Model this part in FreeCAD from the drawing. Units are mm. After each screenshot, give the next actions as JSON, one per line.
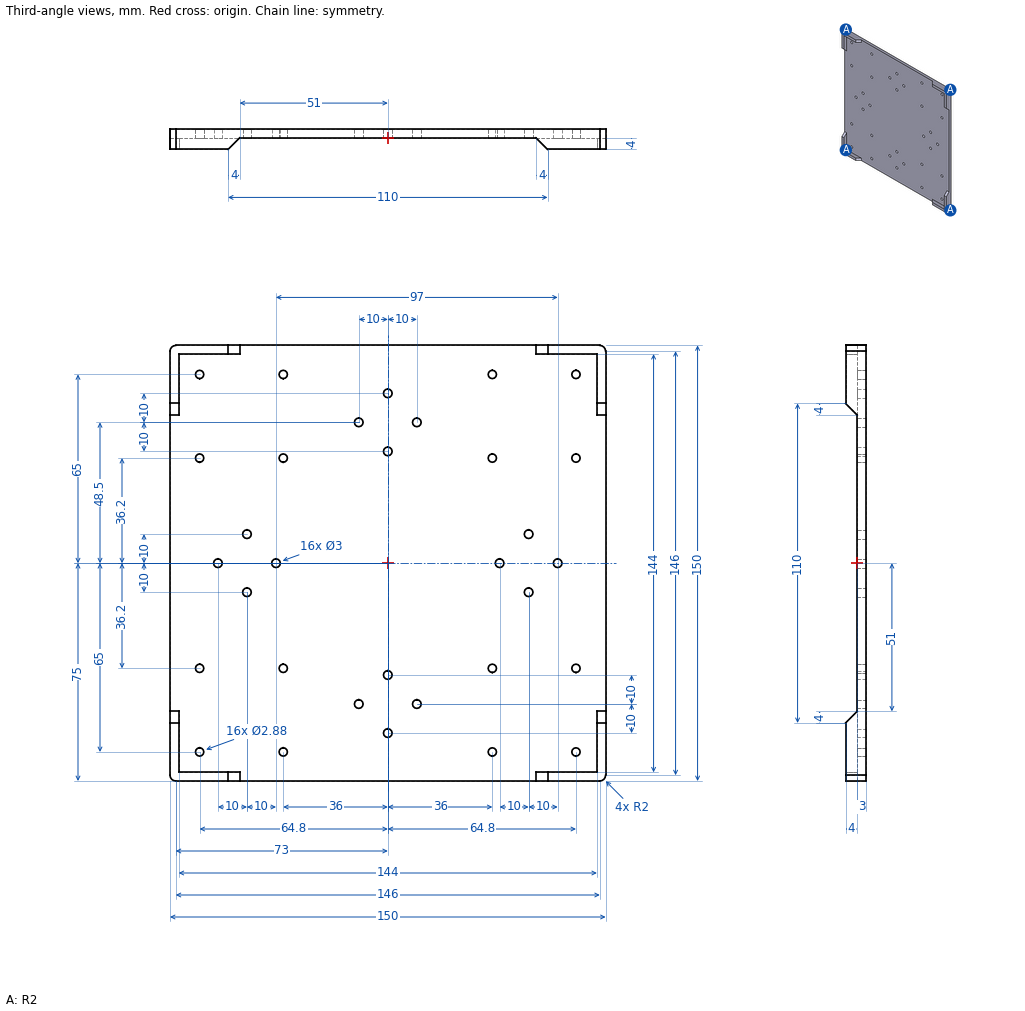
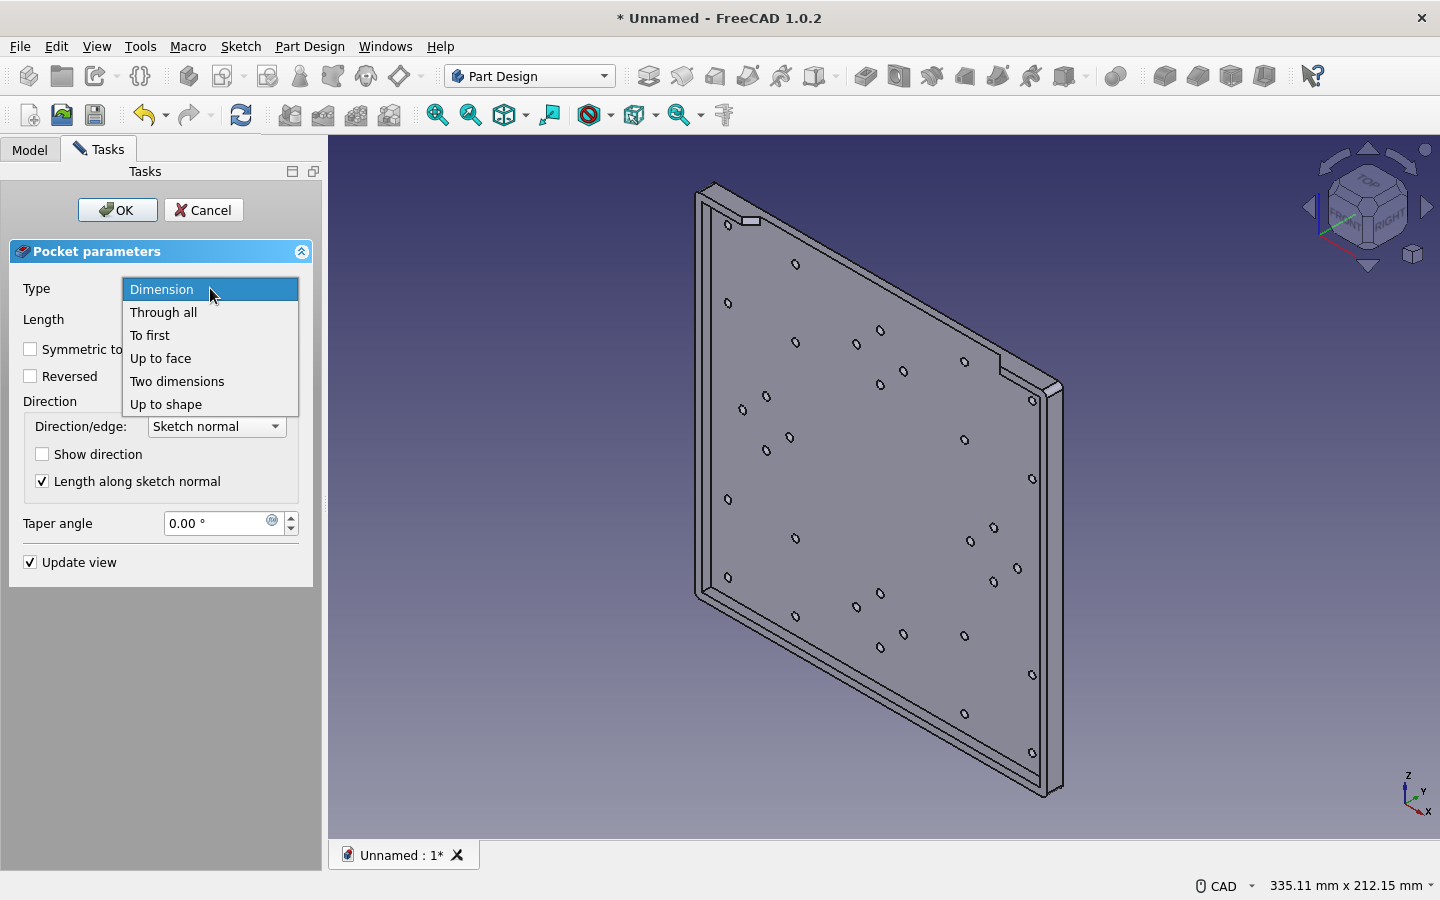
{"action": "left_click", "coordinate": [208, 312]}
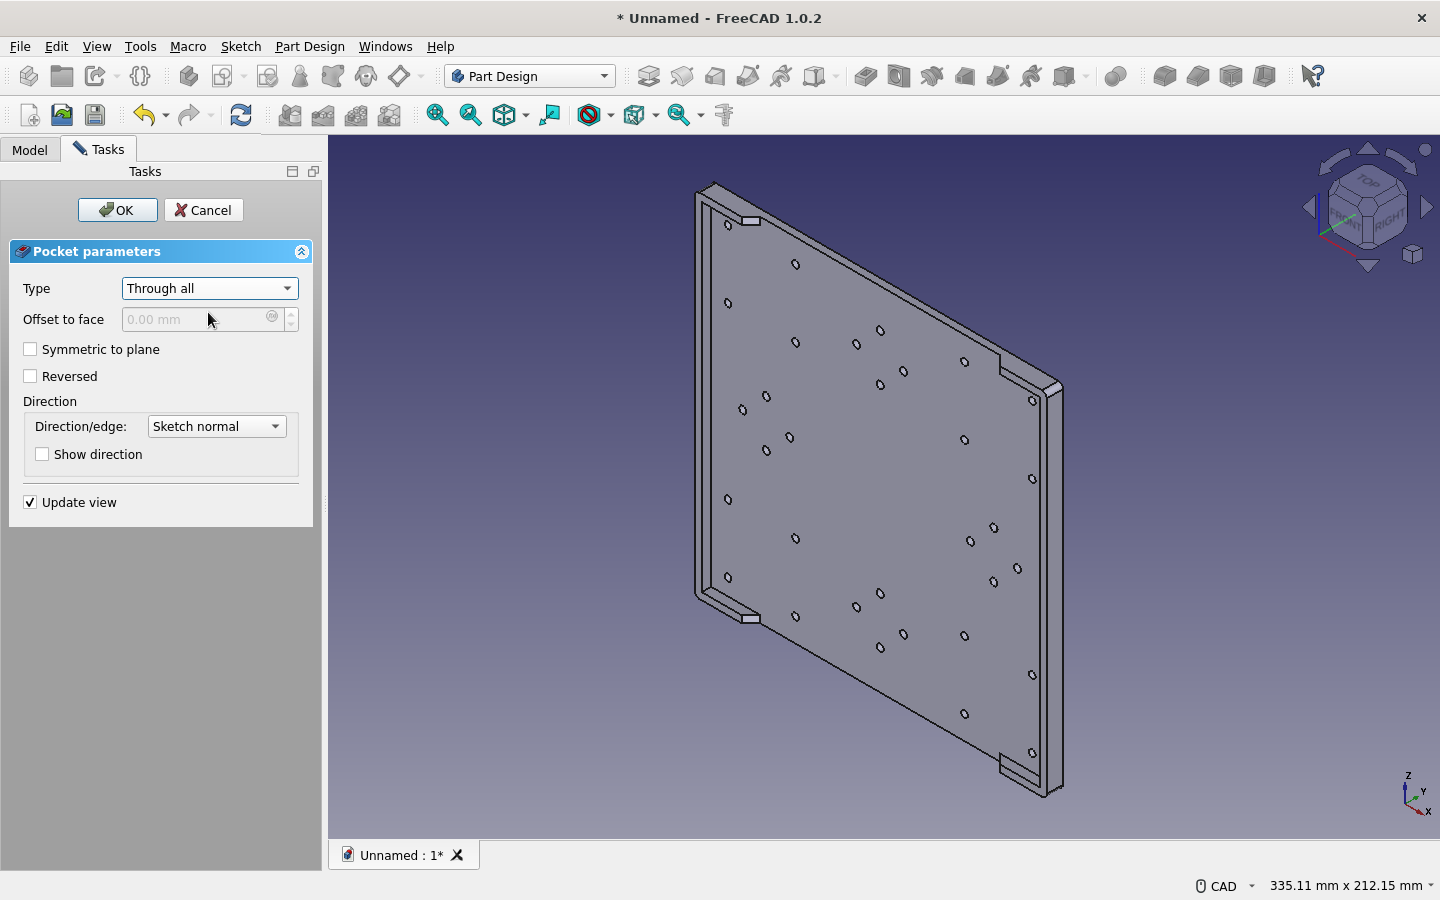
{"action": "left_click", "coordinate": [118, 210]}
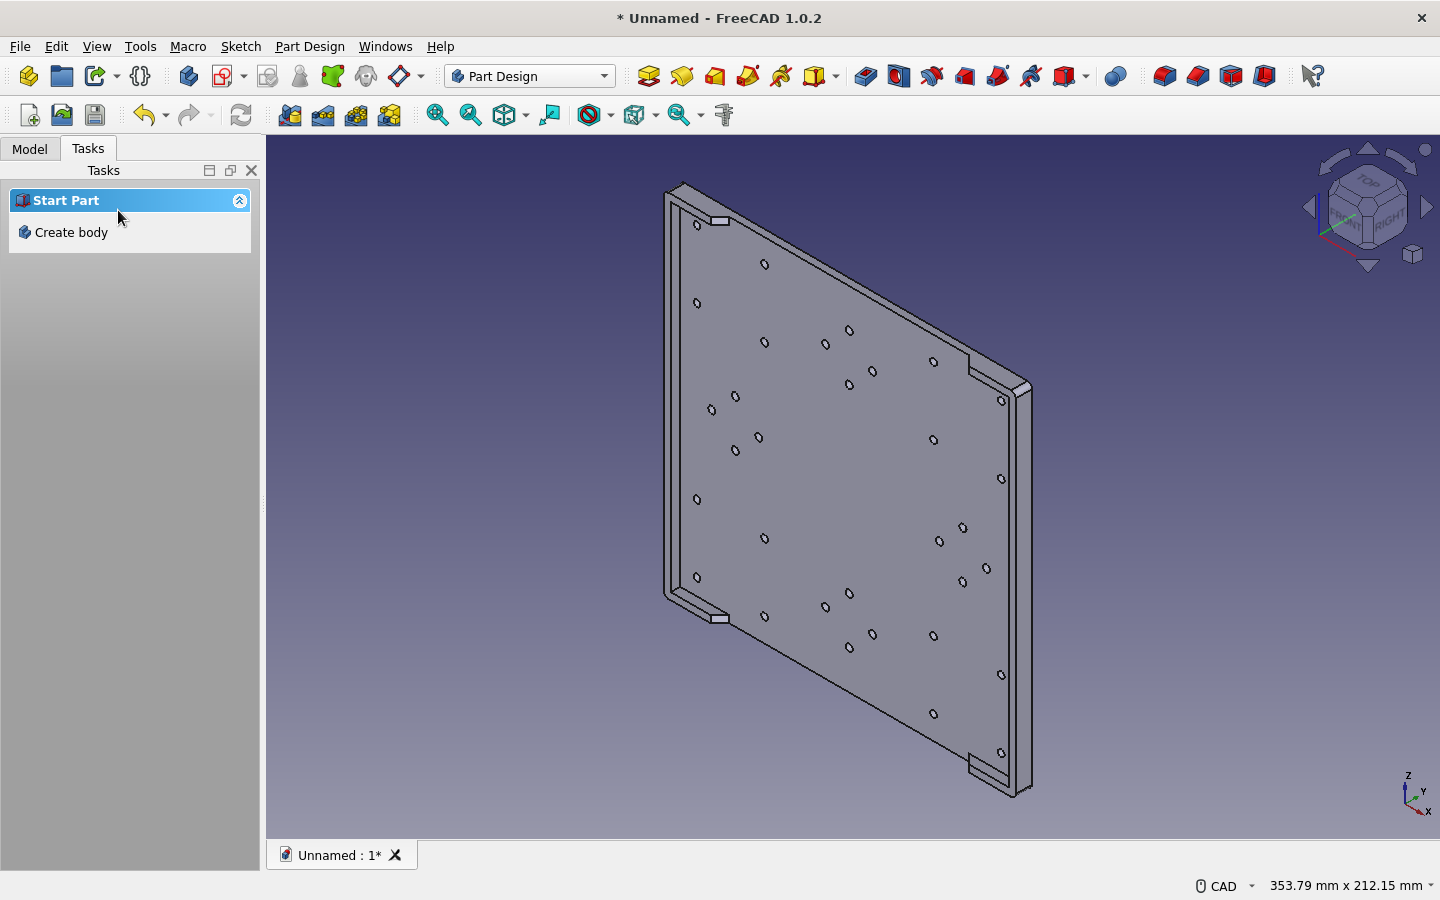
{"action": "key", "text": "6"}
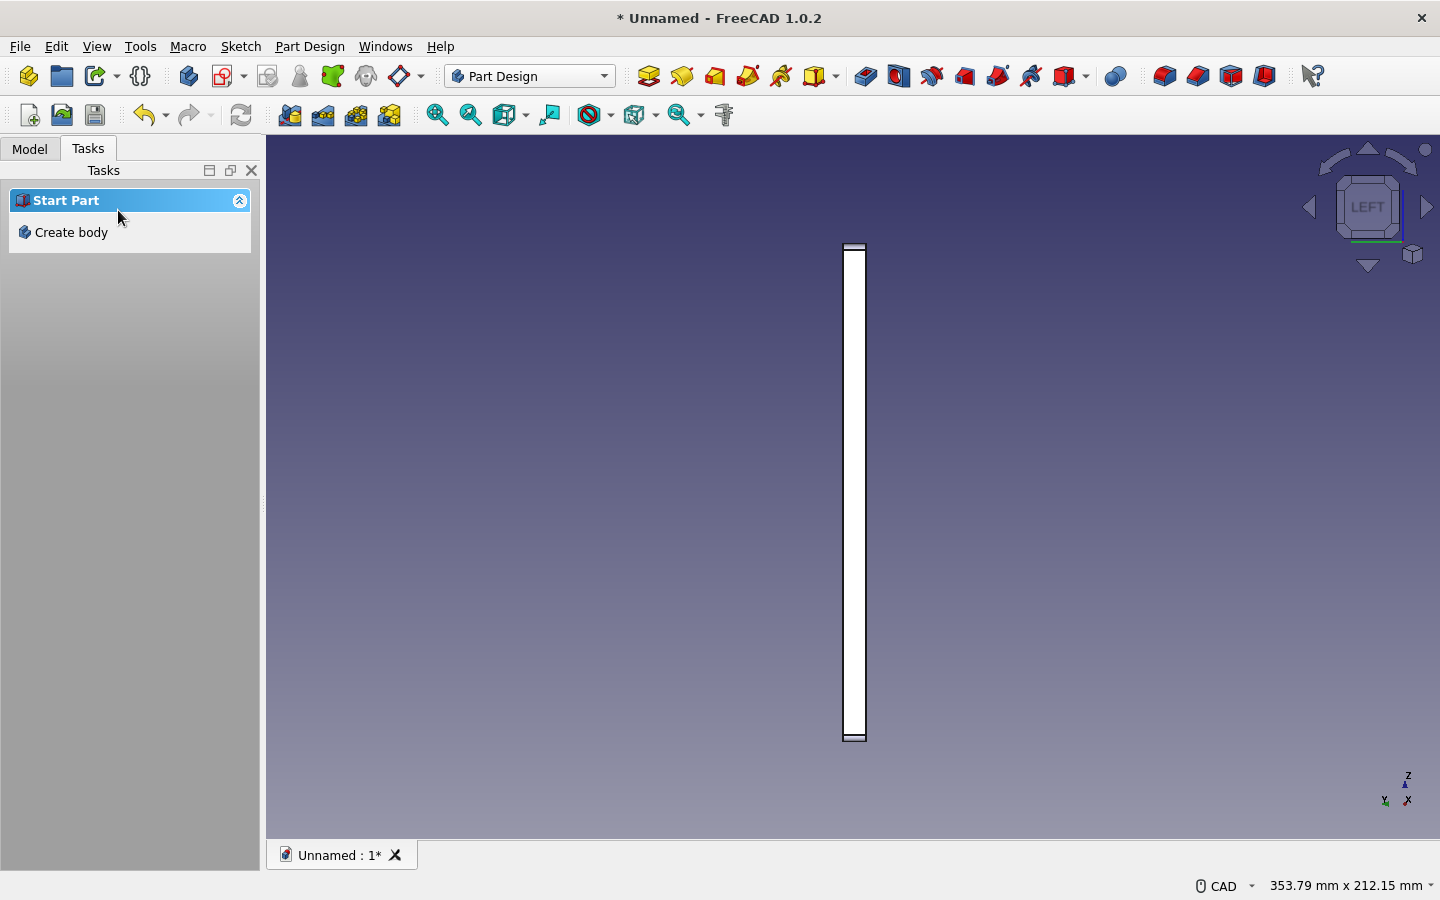
{"action": "left_click", "coordinate": [855, 492]}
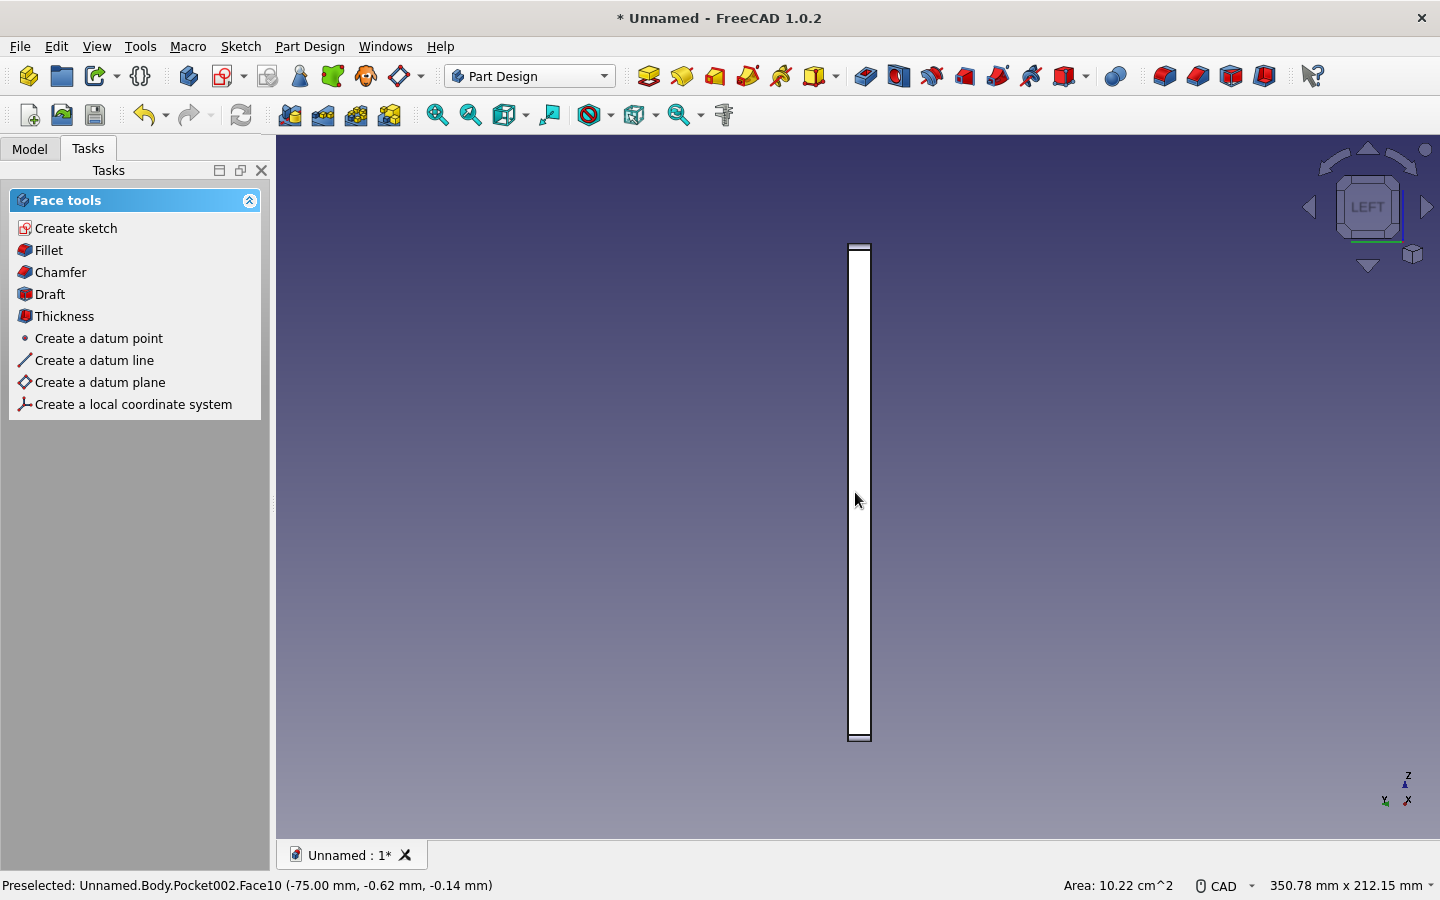
{"action": "left_click", "coordinate": [222, 76]}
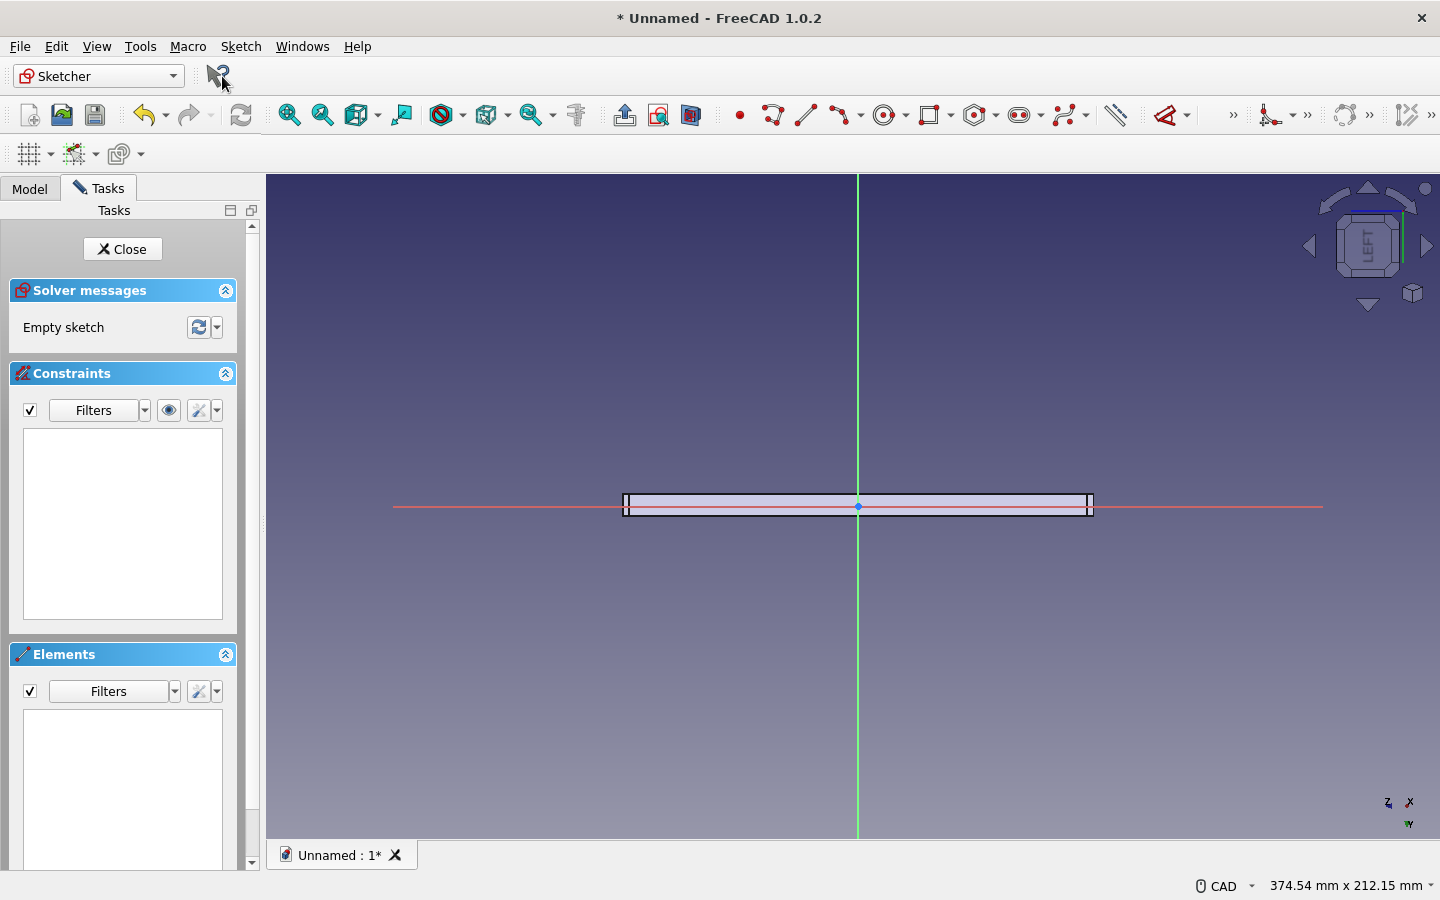
{"action": "scroll", "coordinate": [948, 493], "scroll_direction": "up", "scroll_amount": 3}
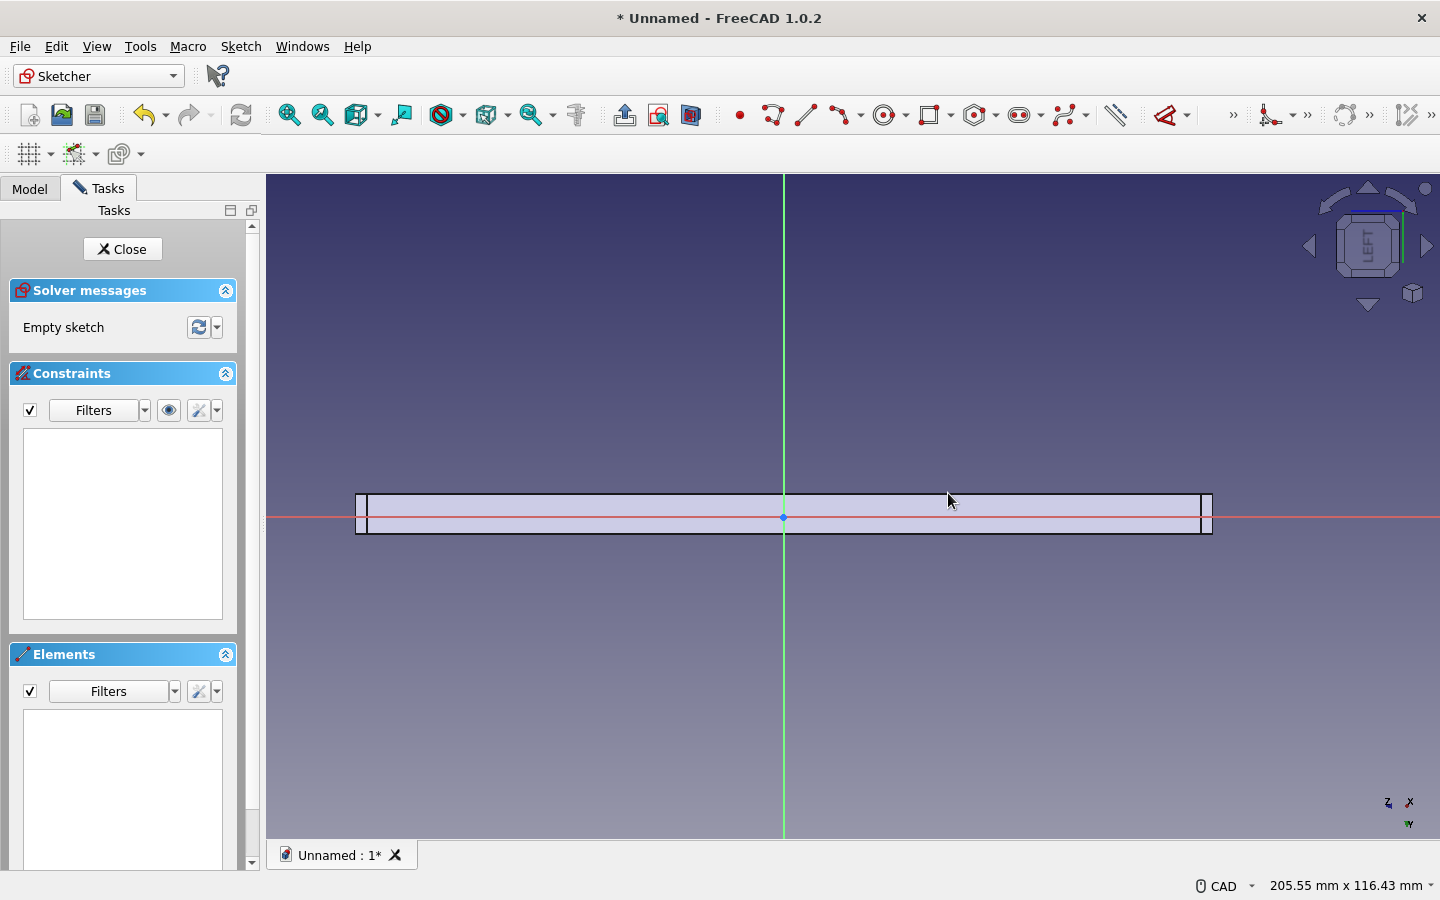
{"action": "key", "text": "g m"}